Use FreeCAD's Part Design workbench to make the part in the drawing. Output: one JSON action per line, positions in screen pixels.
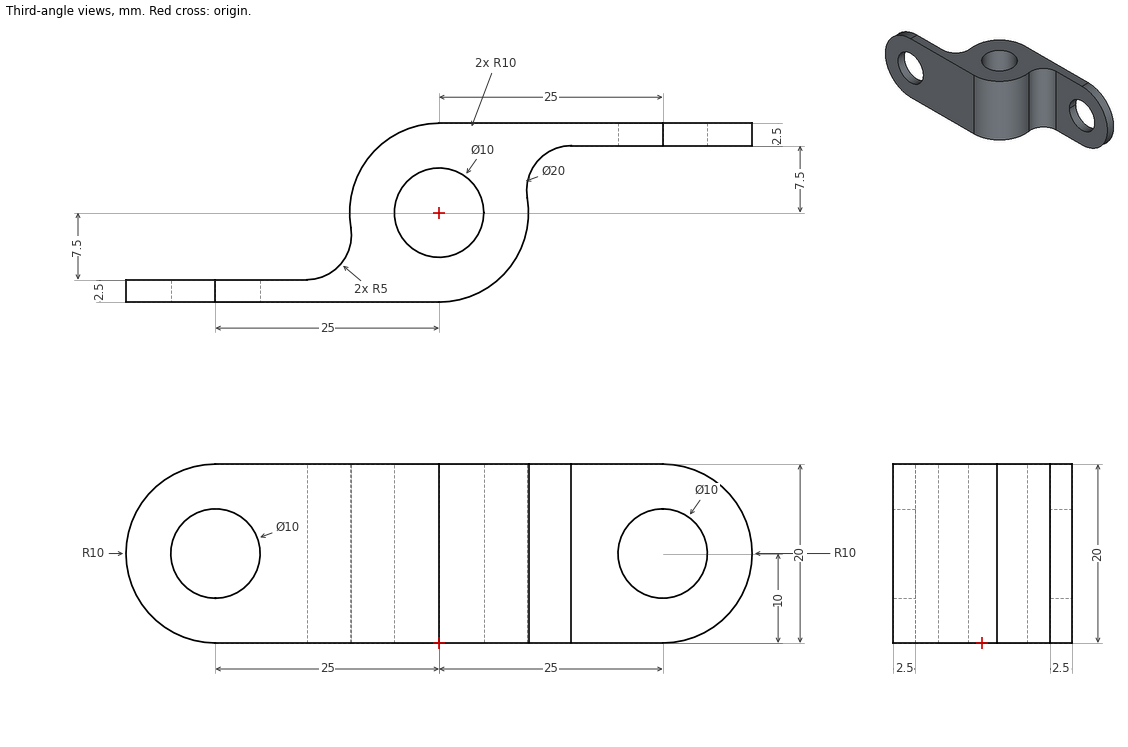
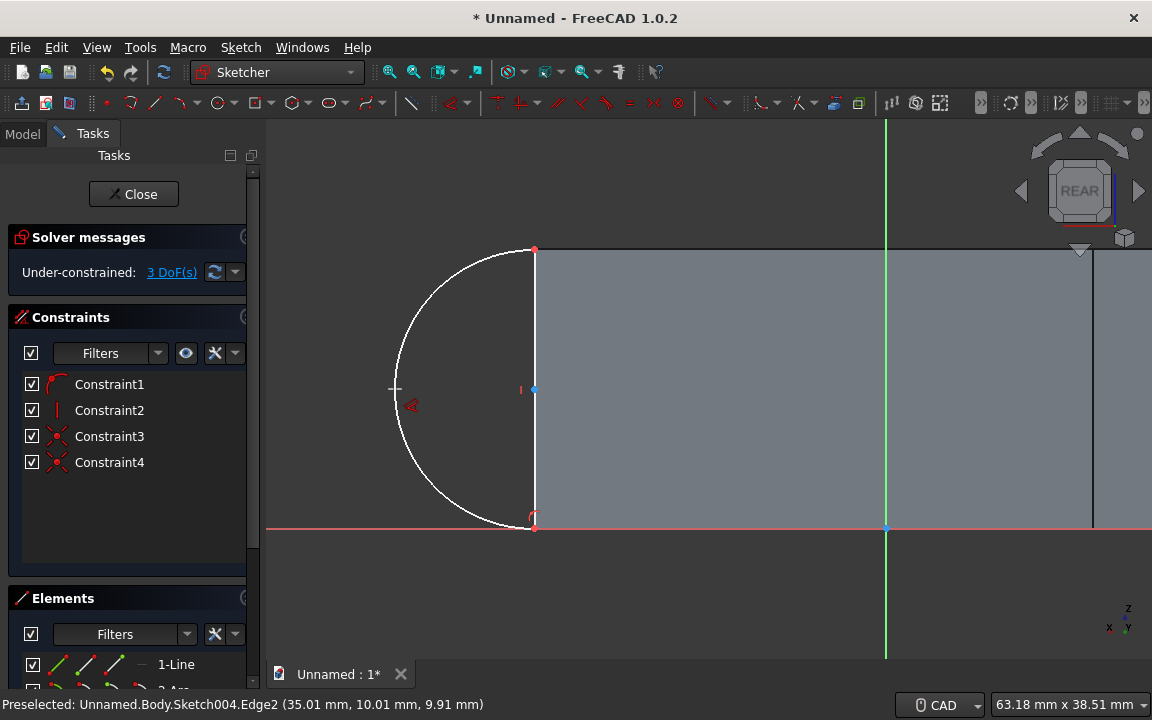
{"action": "left_click", "coordinate": [422, 307]}
{"action": "left_click", "coordinate": [396, 288]}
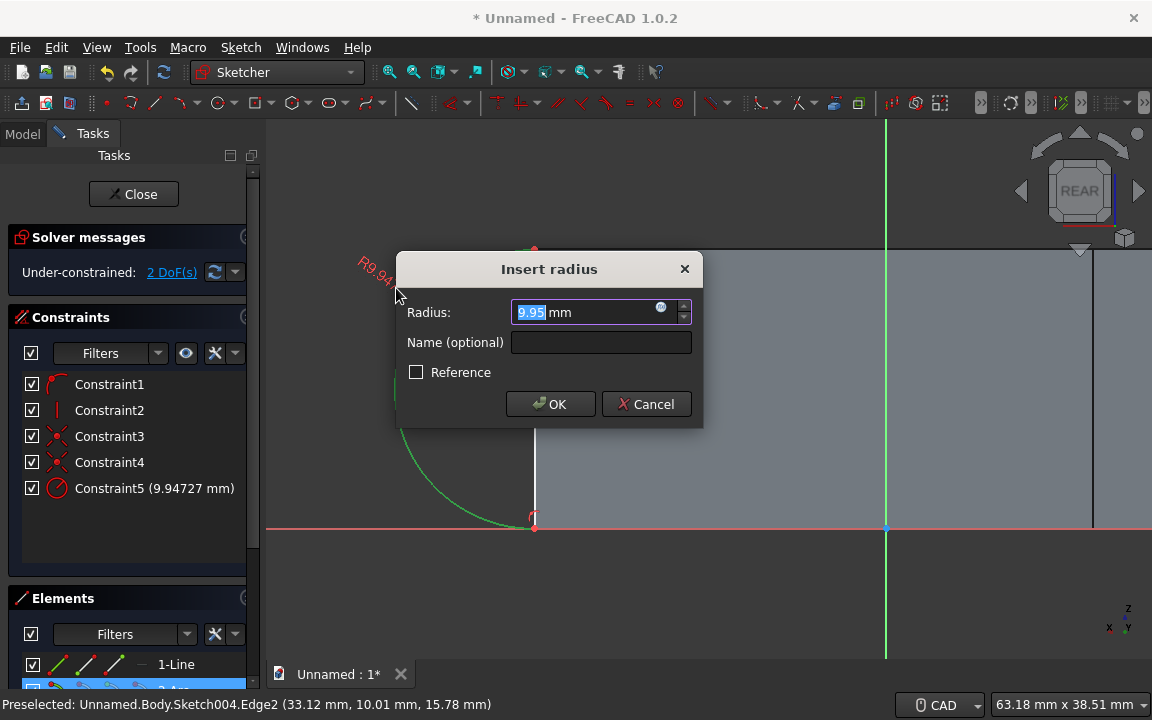
{"action": "type", "text": "10"}
{"action": "key", "text": "Return"}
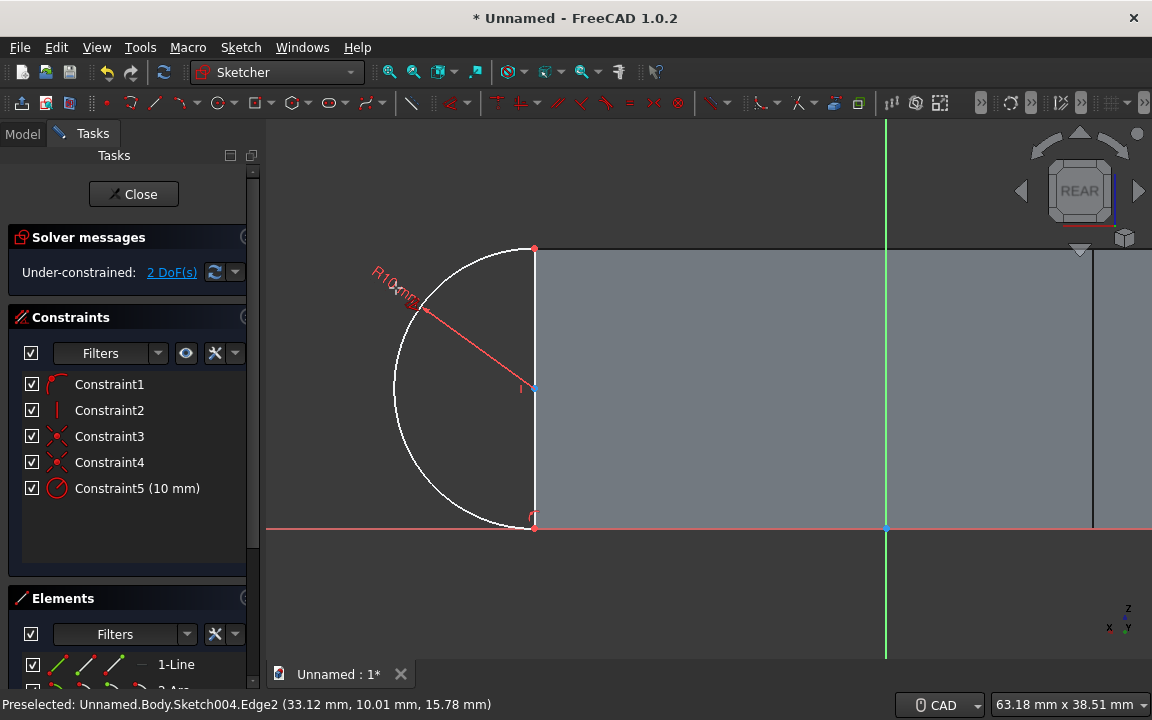
{"action": "left_click", "coordinate": [535, 529]}
{"action": "left_click", "coordinate": [711, 563]}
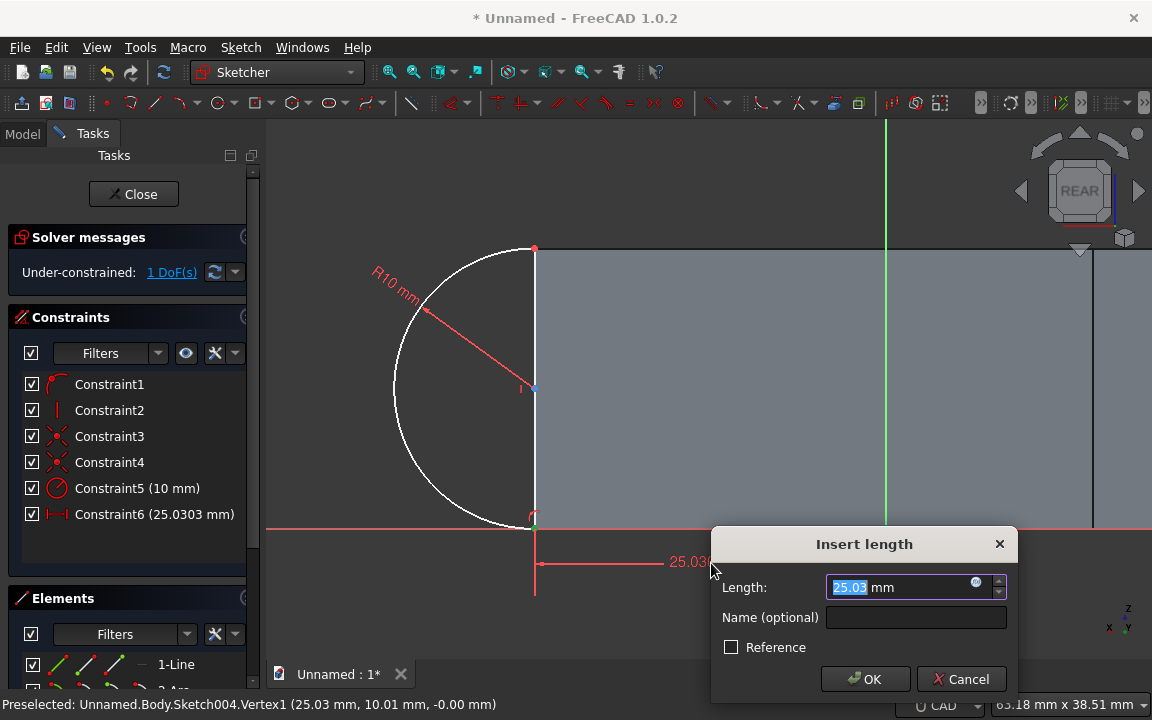
{"action": "type", "text": "25"}
{"action": "key", "text": "Return"}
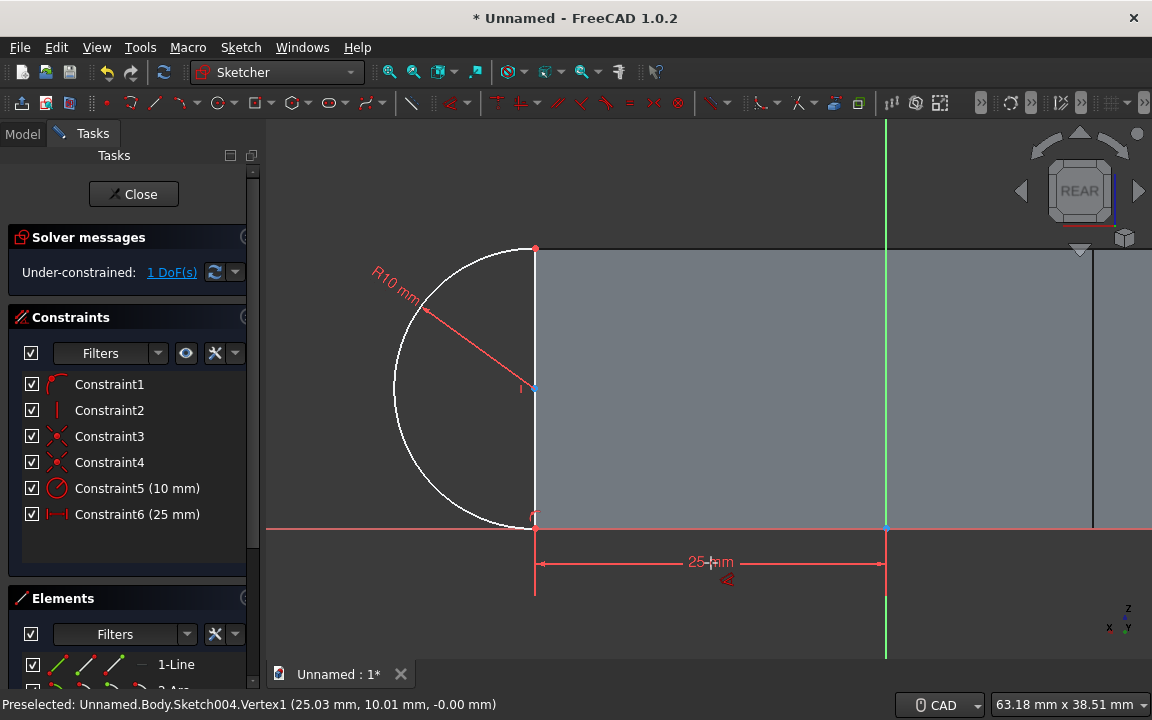
{"action": "left_click", "coordinate": [534, 389]}
{"action": "left_click", "coordinate": [629, 563]}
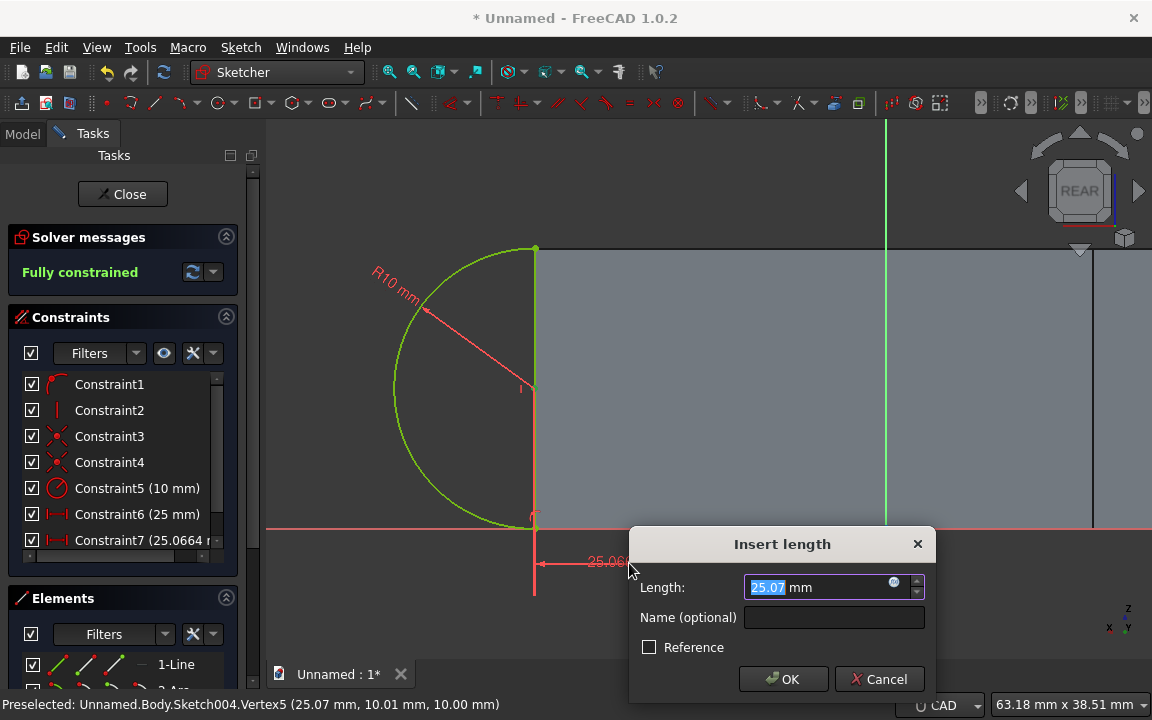
{"action": "type", "text": "25"}
{"action": "key", "text": "Return"}
{"action": "key", "text": "Escape"}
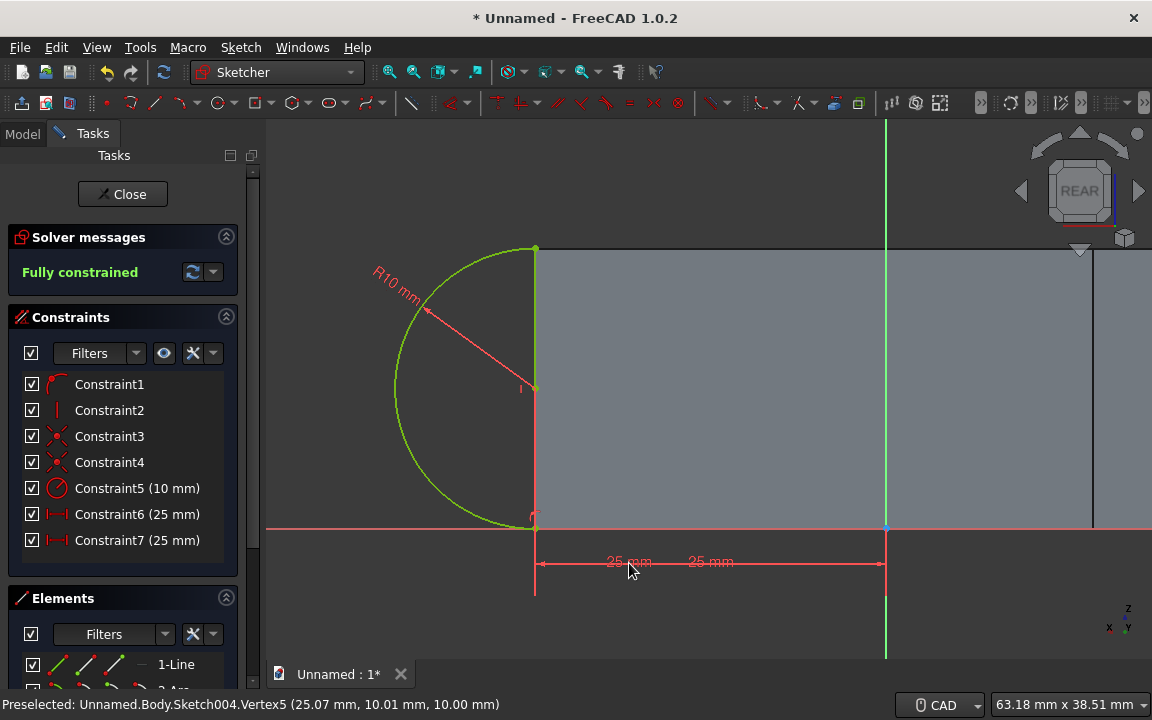
{"action": "left_click", "coordinate": [123, 194]}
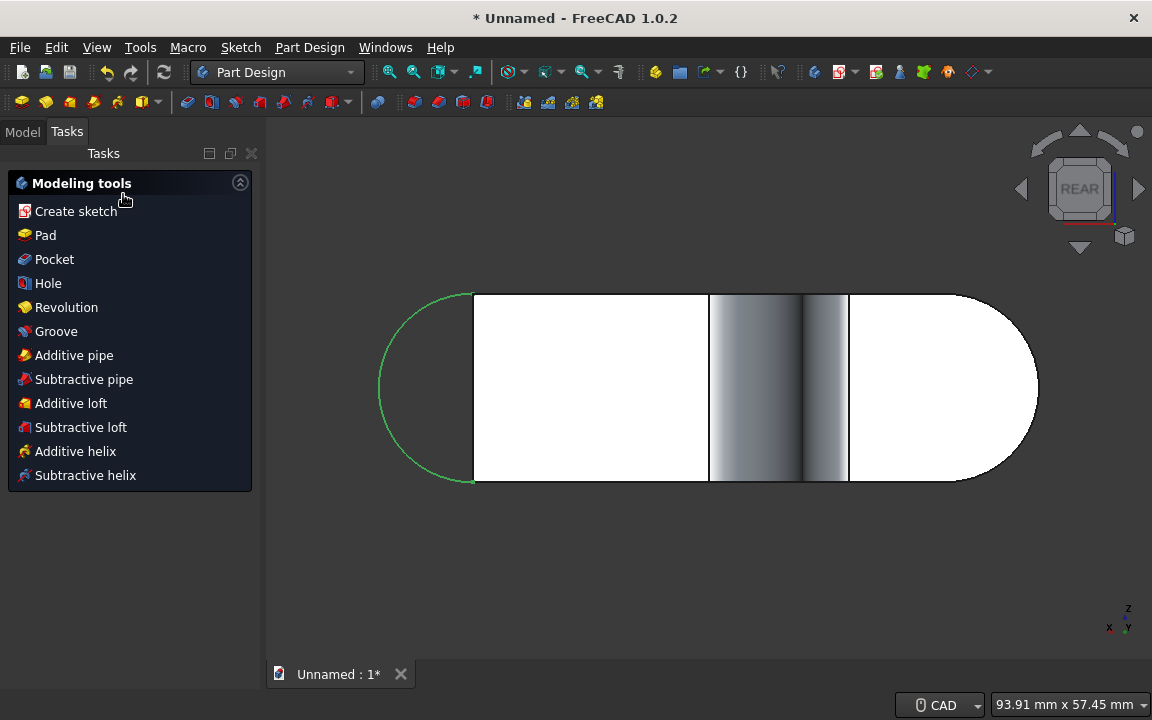
{"action": "left_click", "coordinate": [22, 102]}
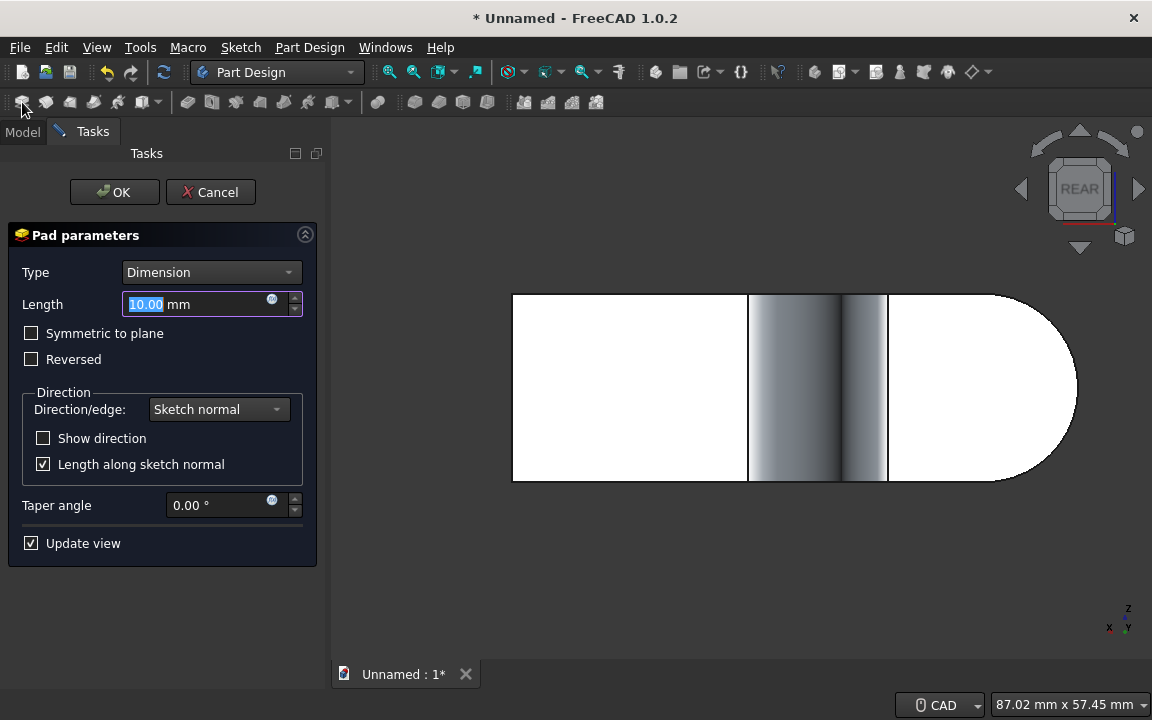
{"action": "type", "text": "2.5"}
{"action": "key", "text": "Tab"}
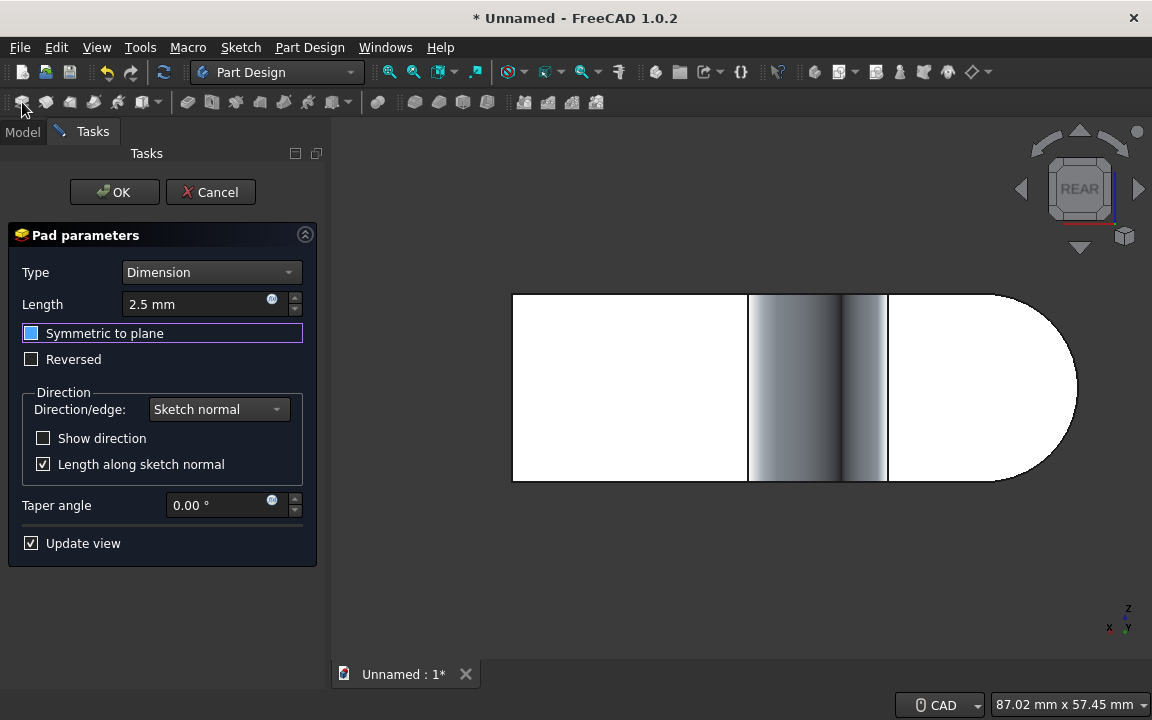
{"action": "left_click", "coordinate": [30, 359]}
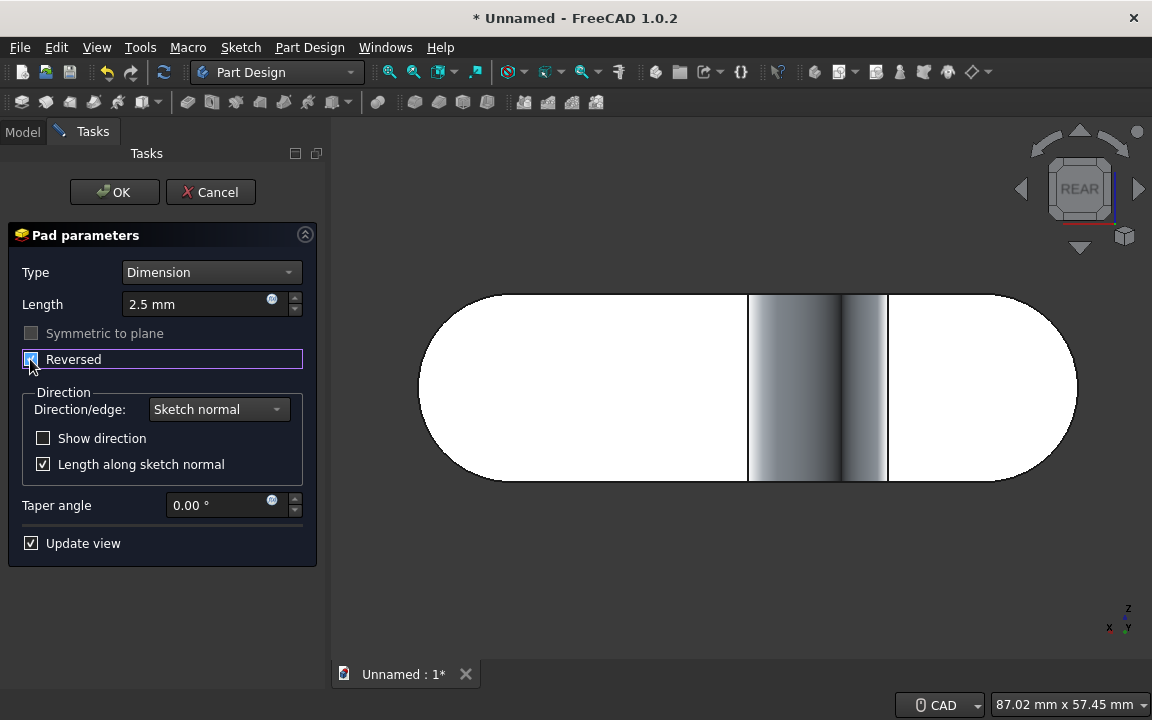
{"action": "left_click", "coordinate": [115, 192]}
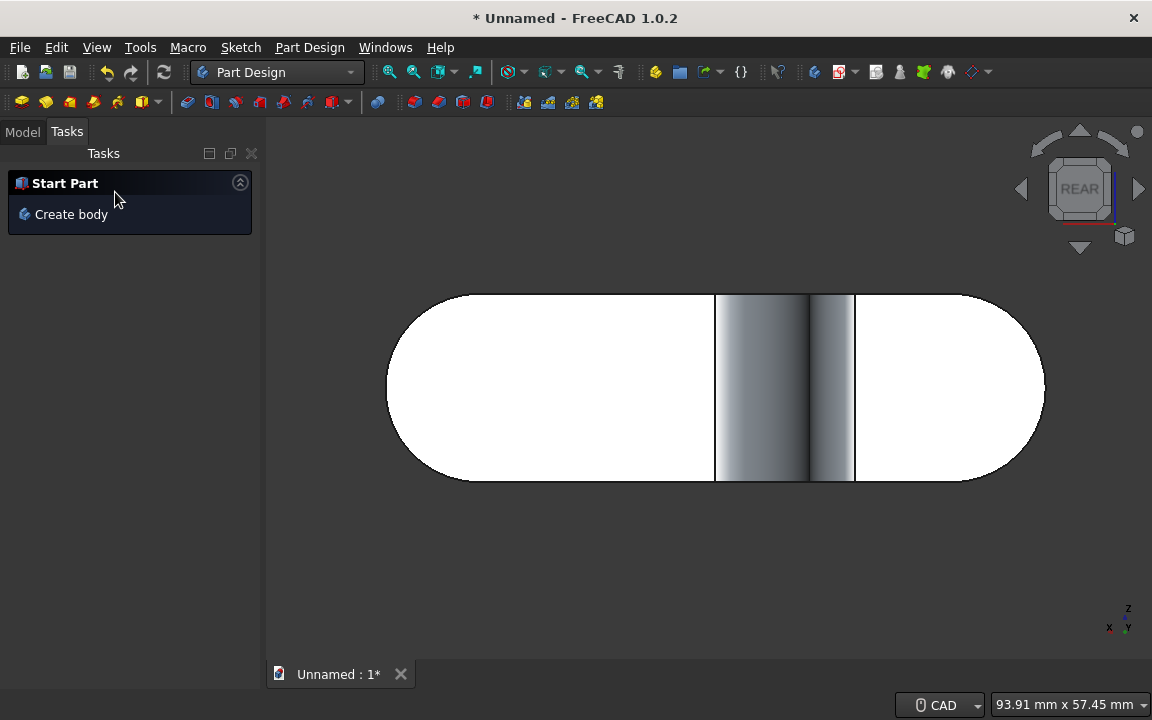
{"action": "left_click", "coordinate": [503, 387]}